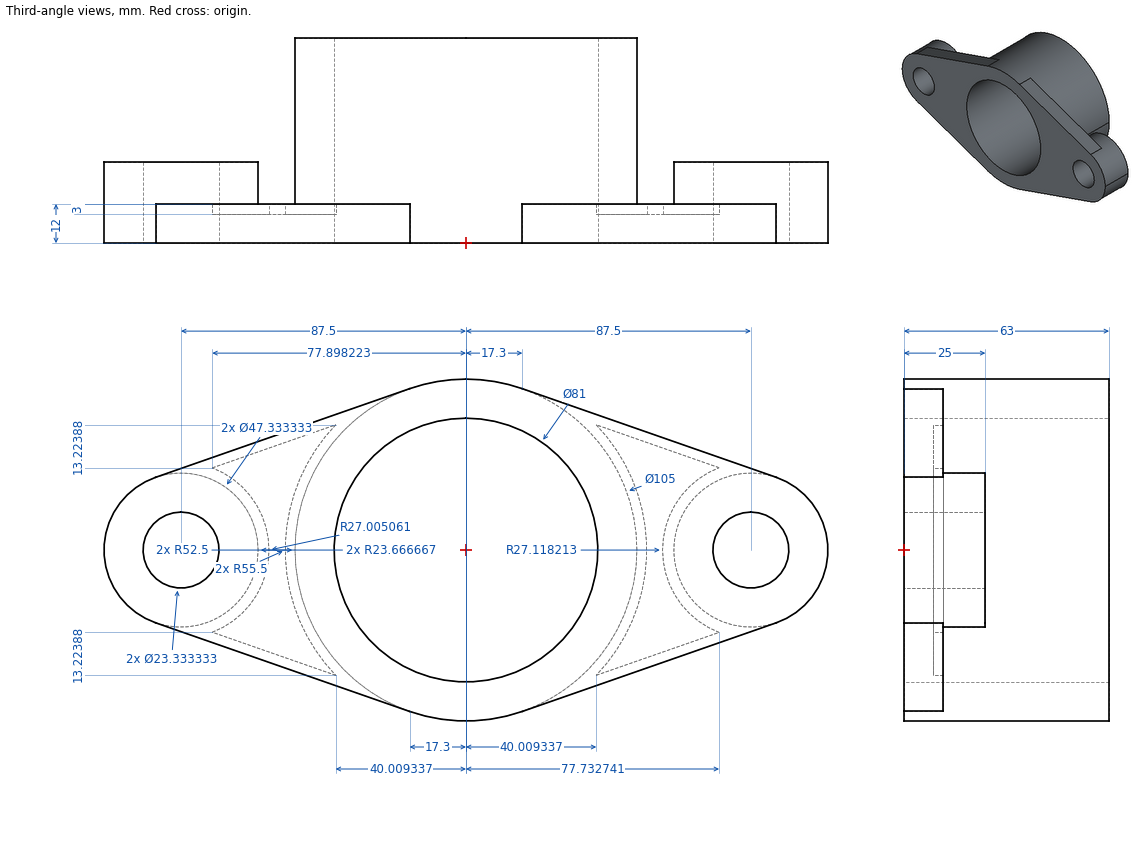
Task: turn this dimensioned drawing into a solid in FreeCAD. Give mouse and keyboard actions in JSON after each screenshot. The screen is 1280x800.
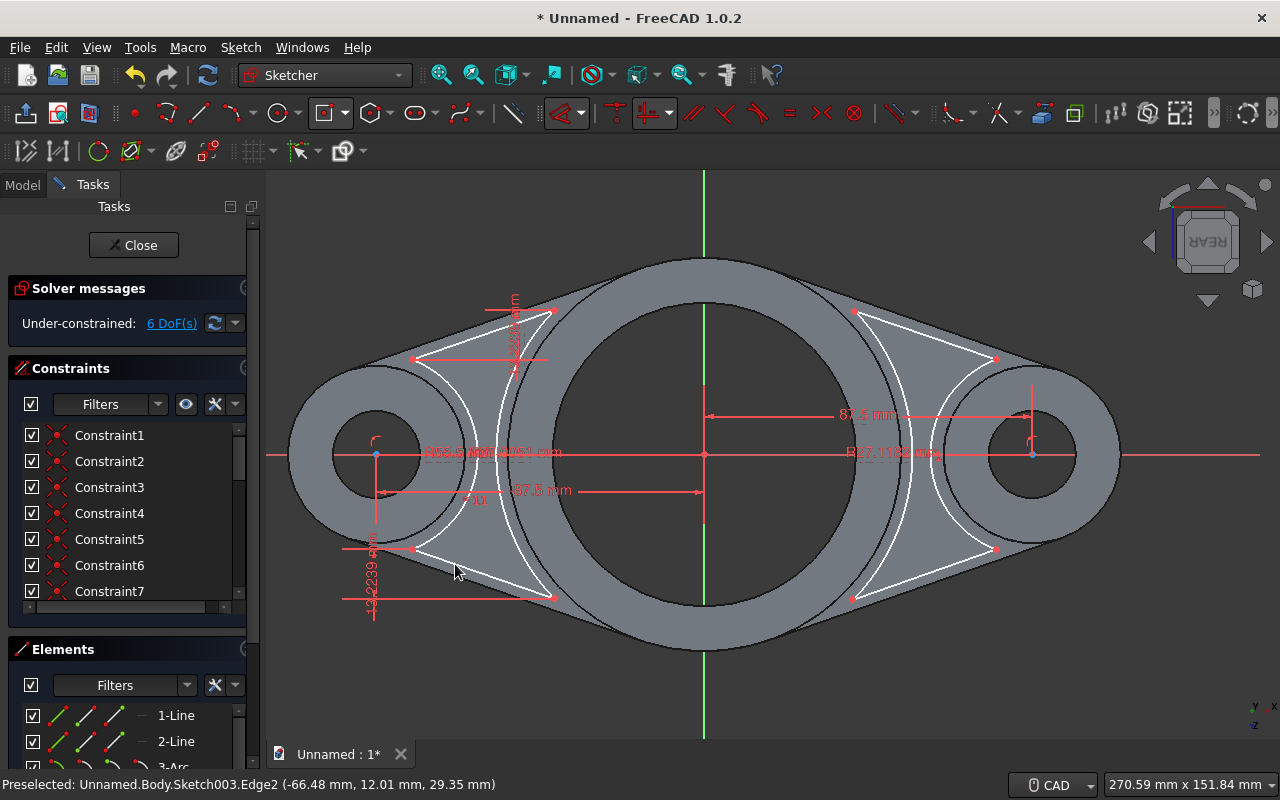
{"action": "left_click", "coordinate": [555, 310]}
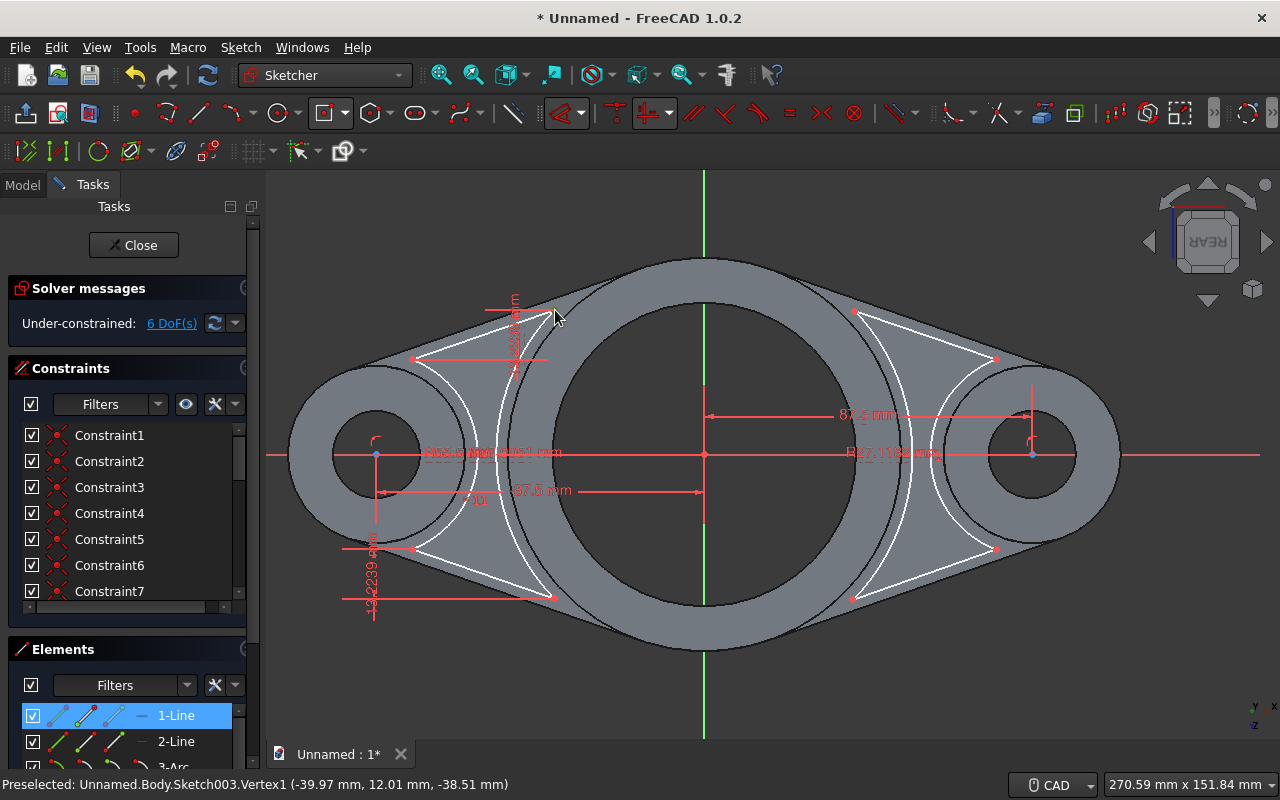
{"action": "key", "text": "l"}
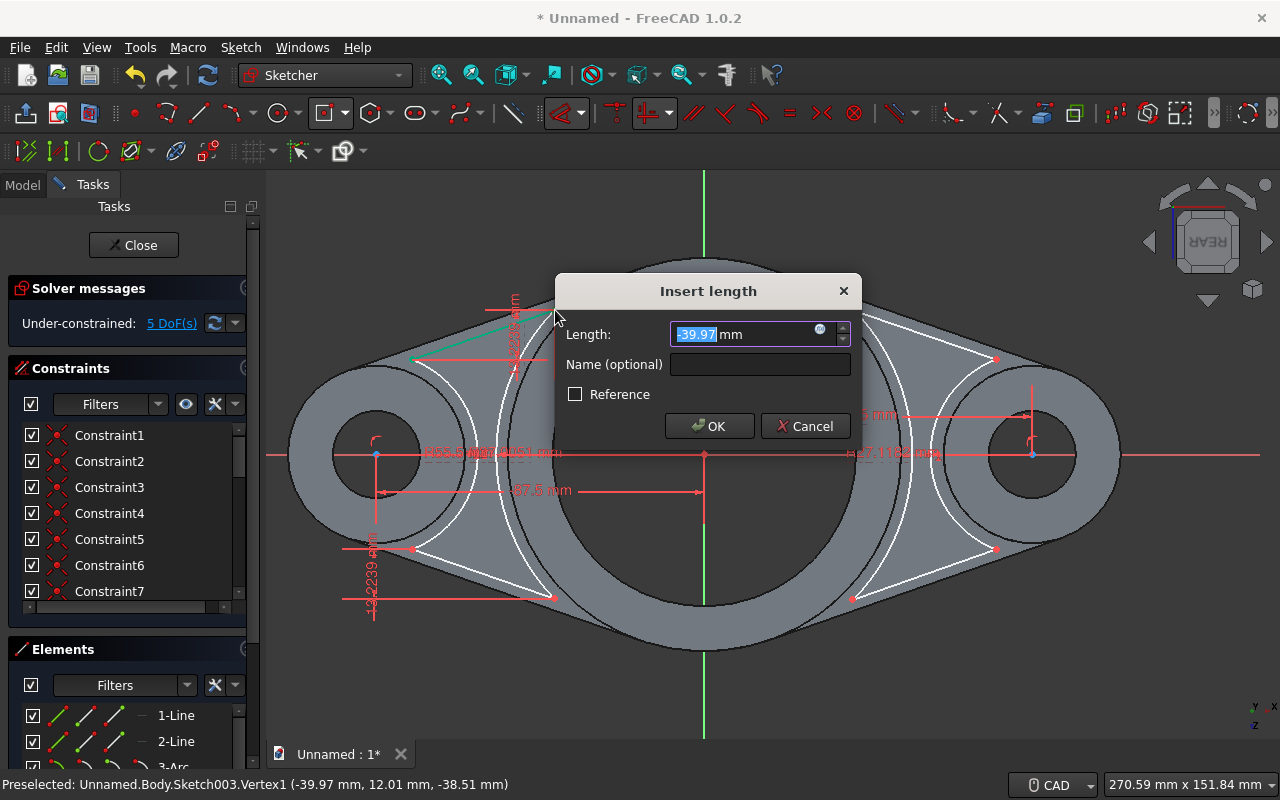
{"action": "type", "text": "-40.009337"}
{"action": "key", "text": "Return"}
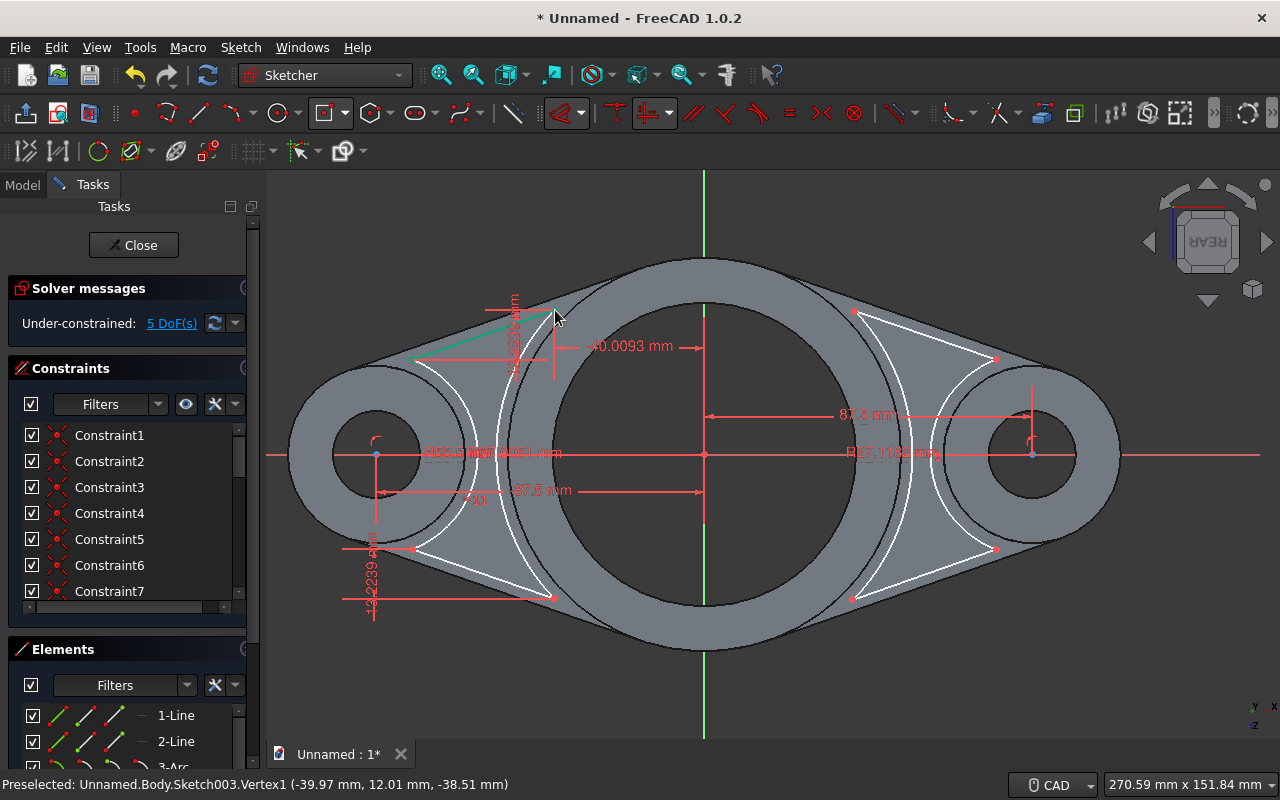
{"action": "left_click", "coordinate": [412, 549]}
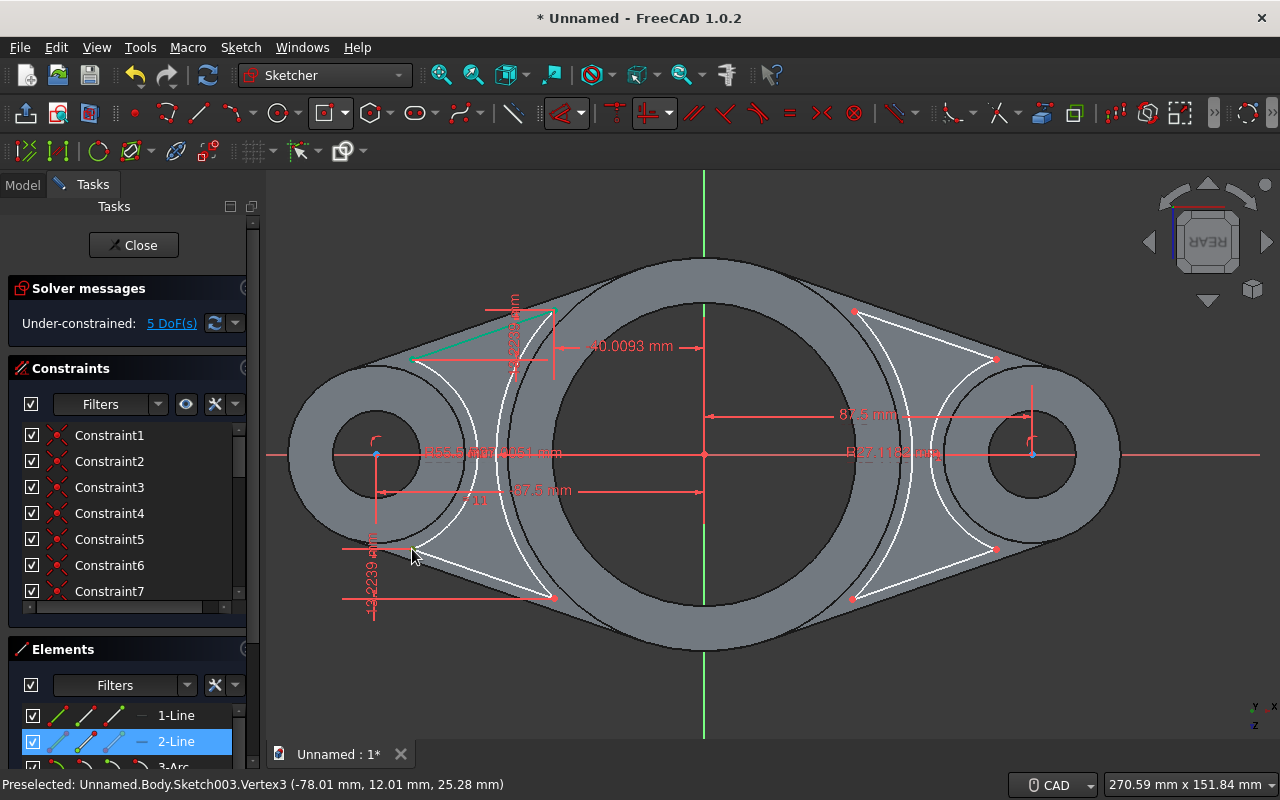
{"action": "left_click", "coordinate": [584, 114]}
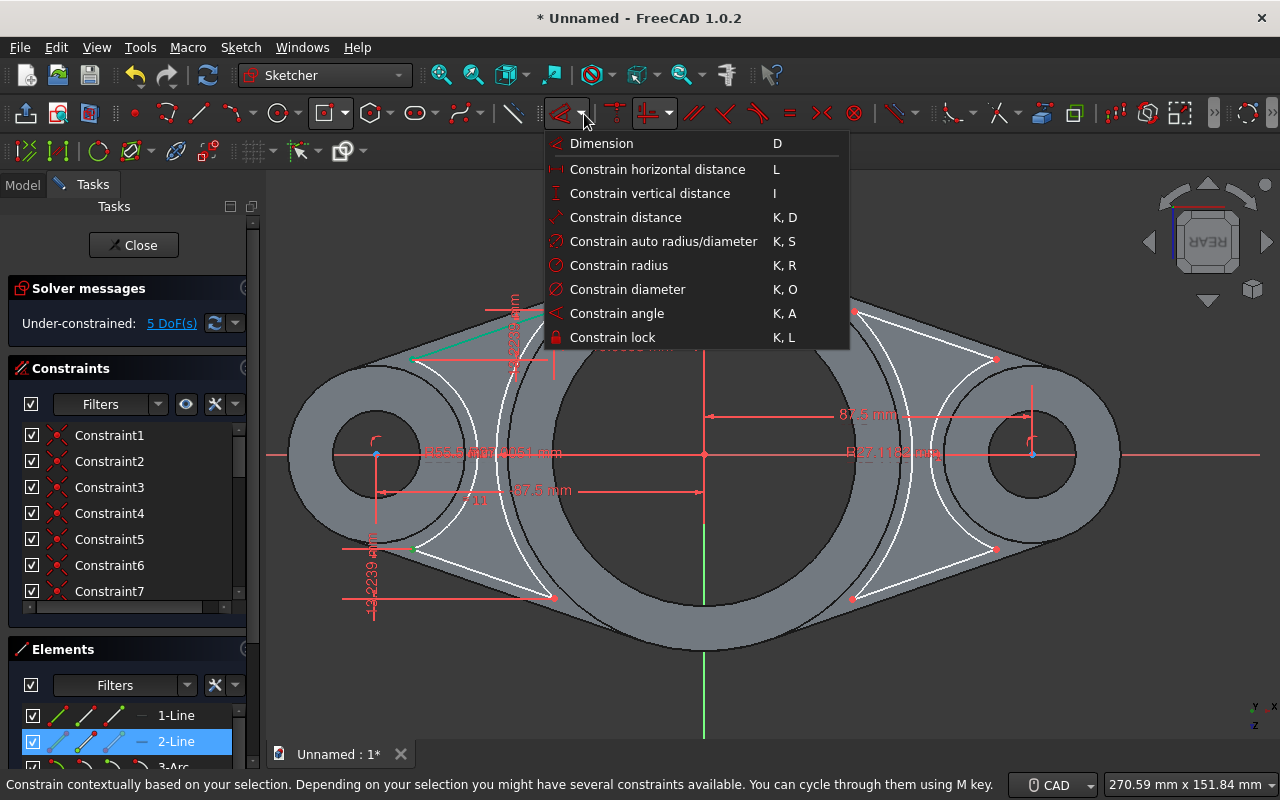
{"action": "left_click", "coordinate": [697, 169]}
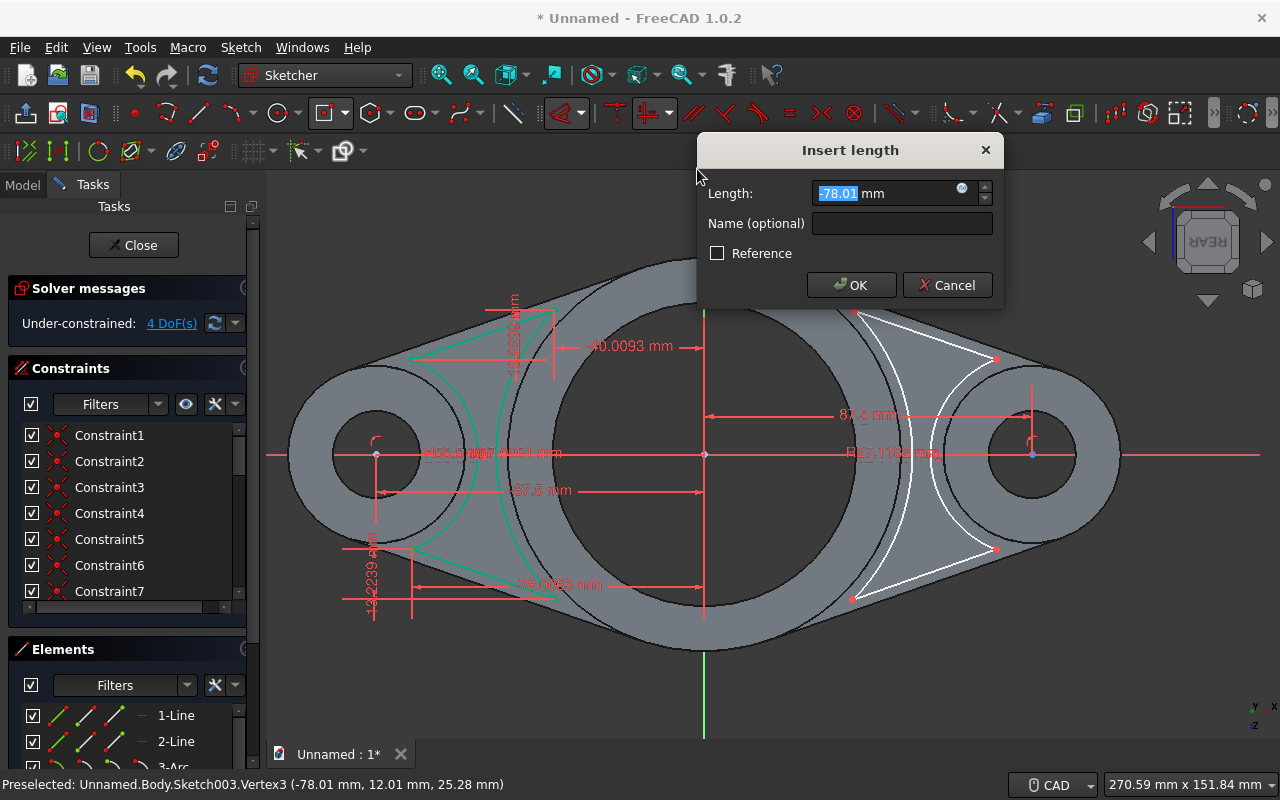
{"action": "type", "text": "-77.898223"}
{"action": "key", "text": "Return"}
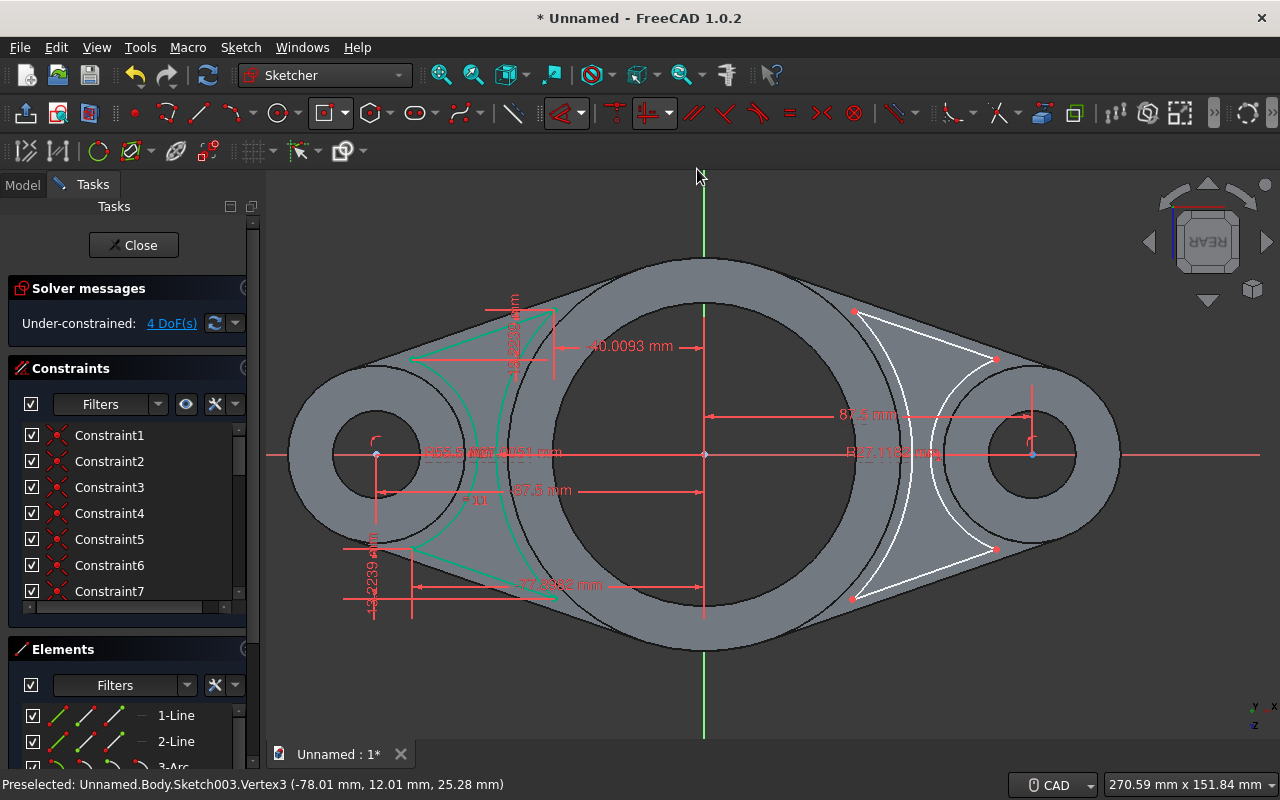
{"action": "left_click", "coordinate": [996, 360]}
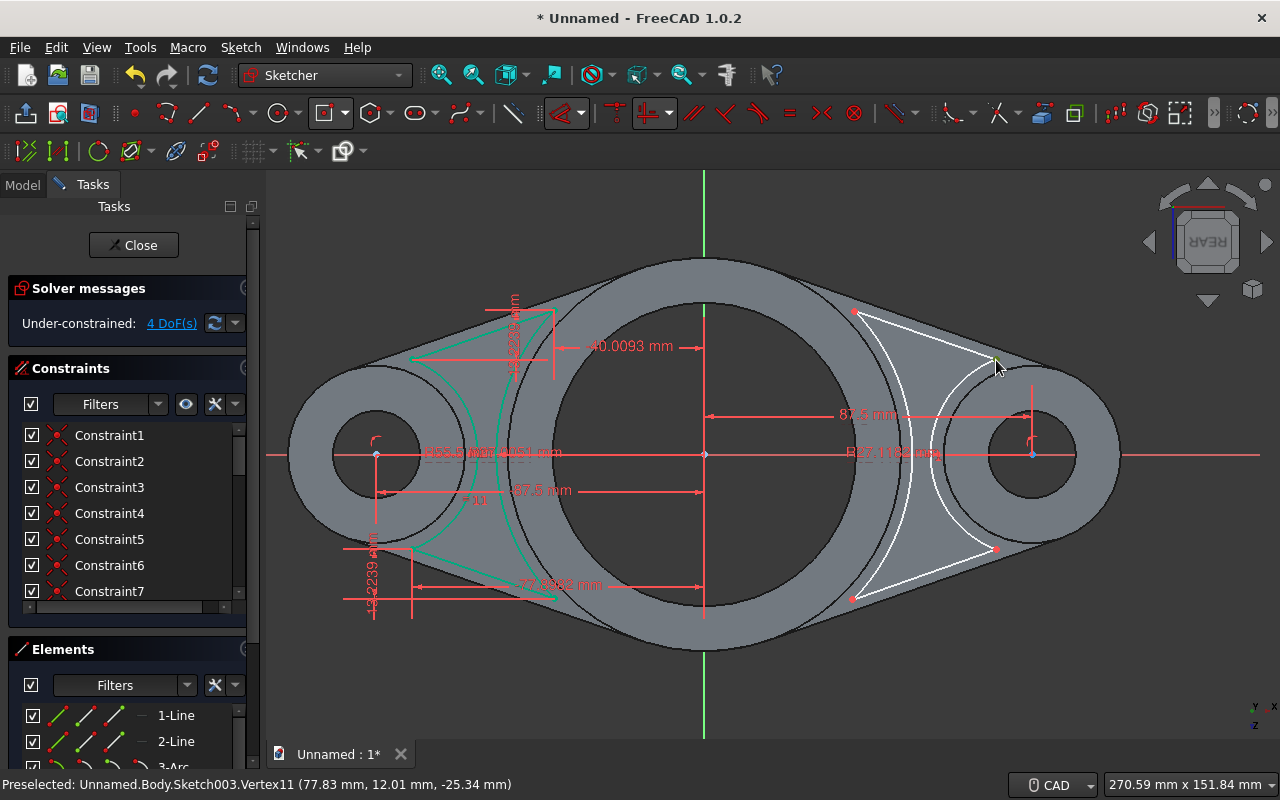
{"action": "key", "text": "l"}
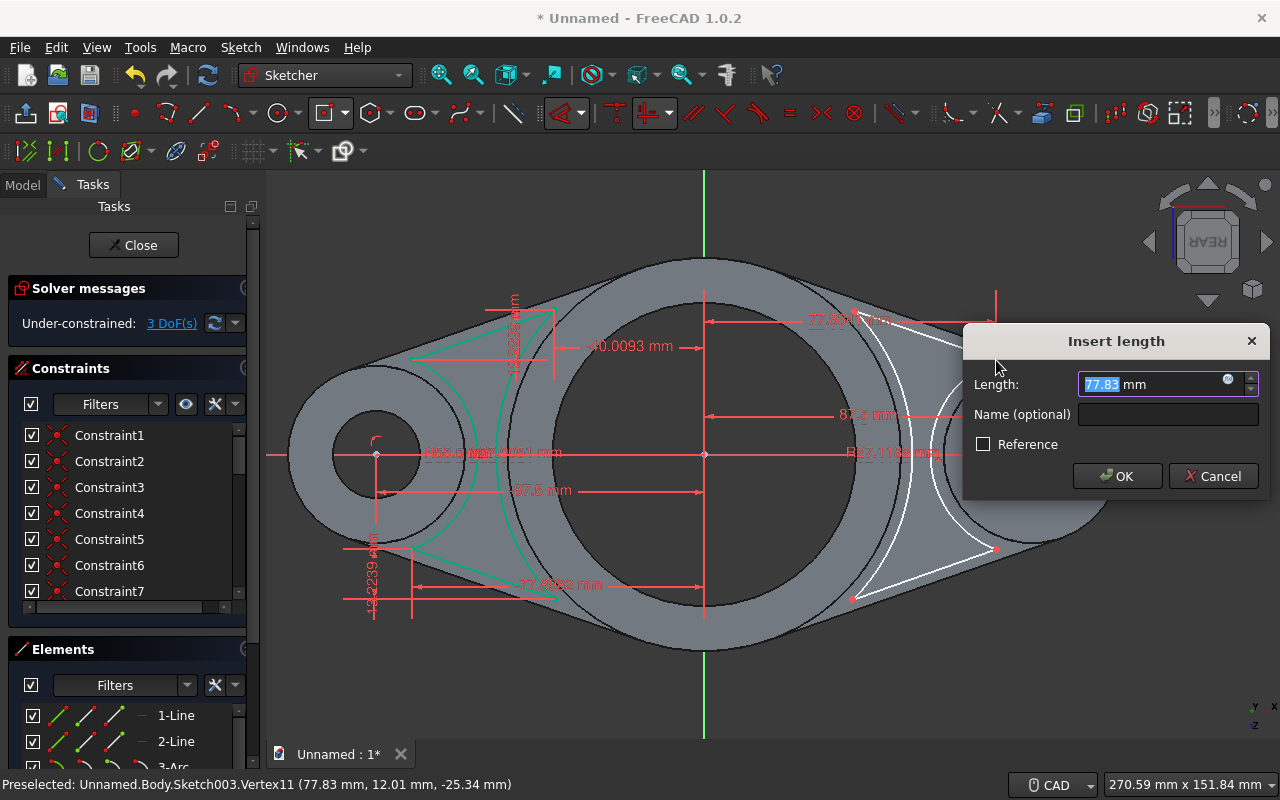
{"action": "type", "text": "77.732741"}
{"action": "key", "text": "Return"}